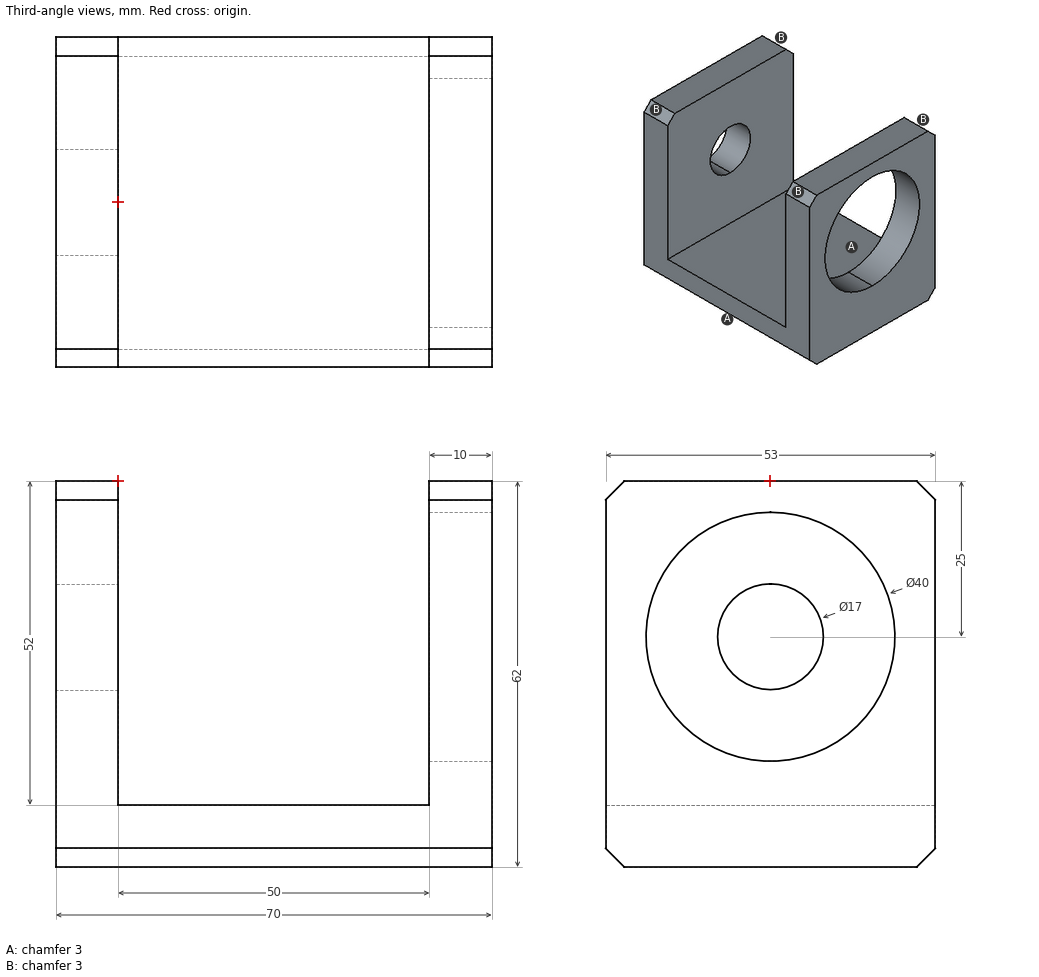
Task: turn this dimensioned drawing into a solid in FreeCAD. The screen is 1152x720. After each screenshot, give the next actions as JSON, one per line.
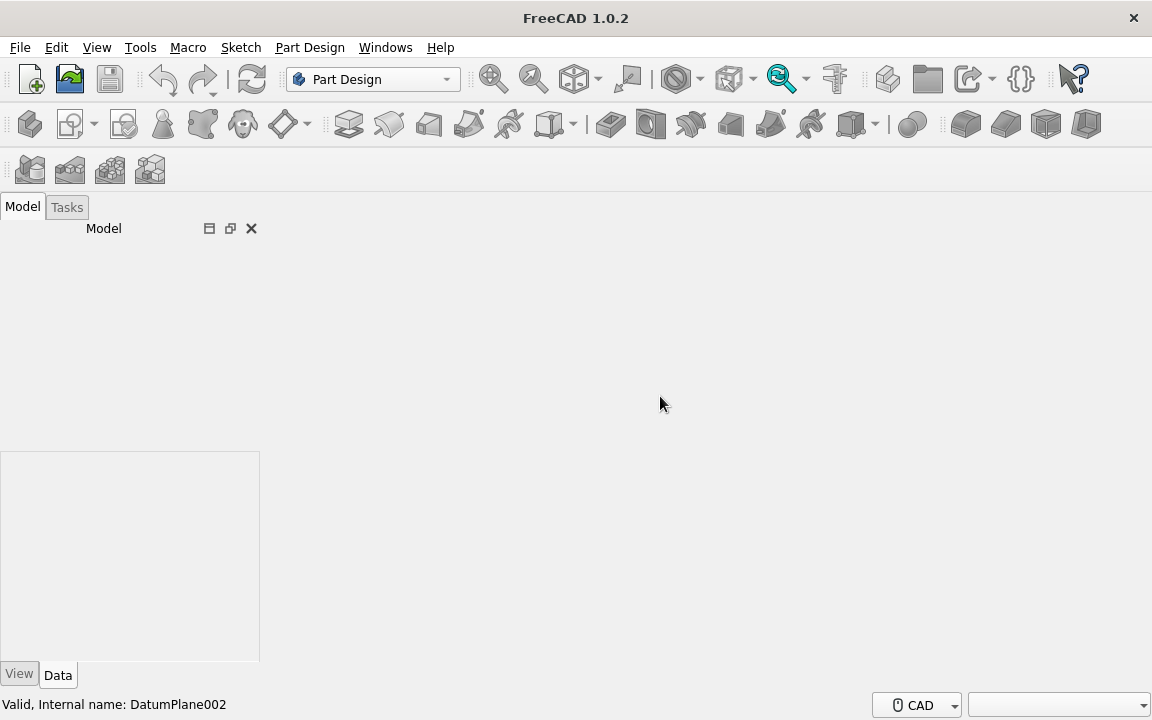
{"action": "key", "text": "ctrl+n"}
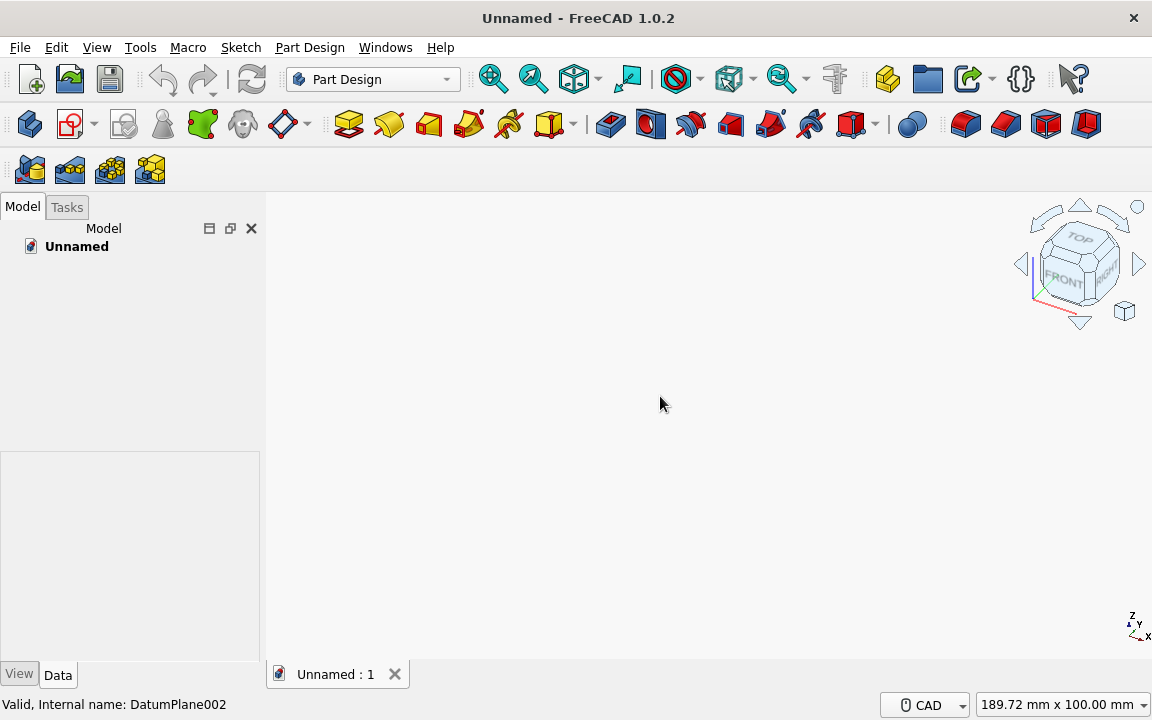
{"action": "left_click", "coordinate": [70, 124]}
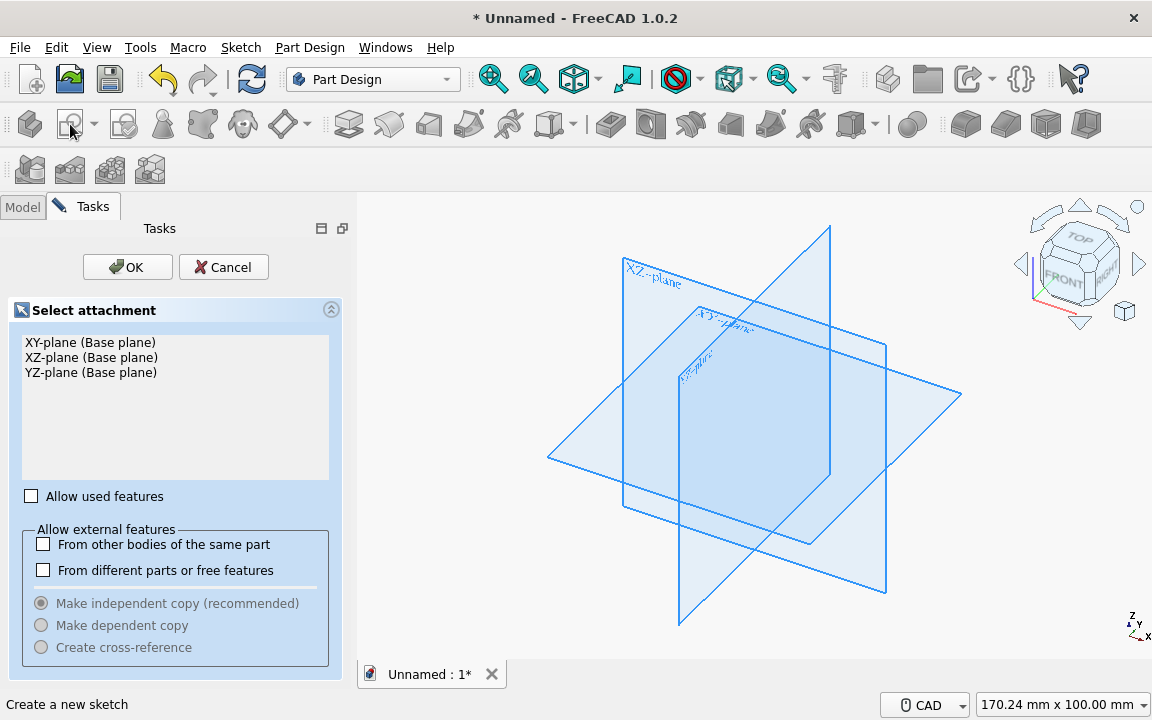
{"action": "left_click", "coordinate": [82, 358]}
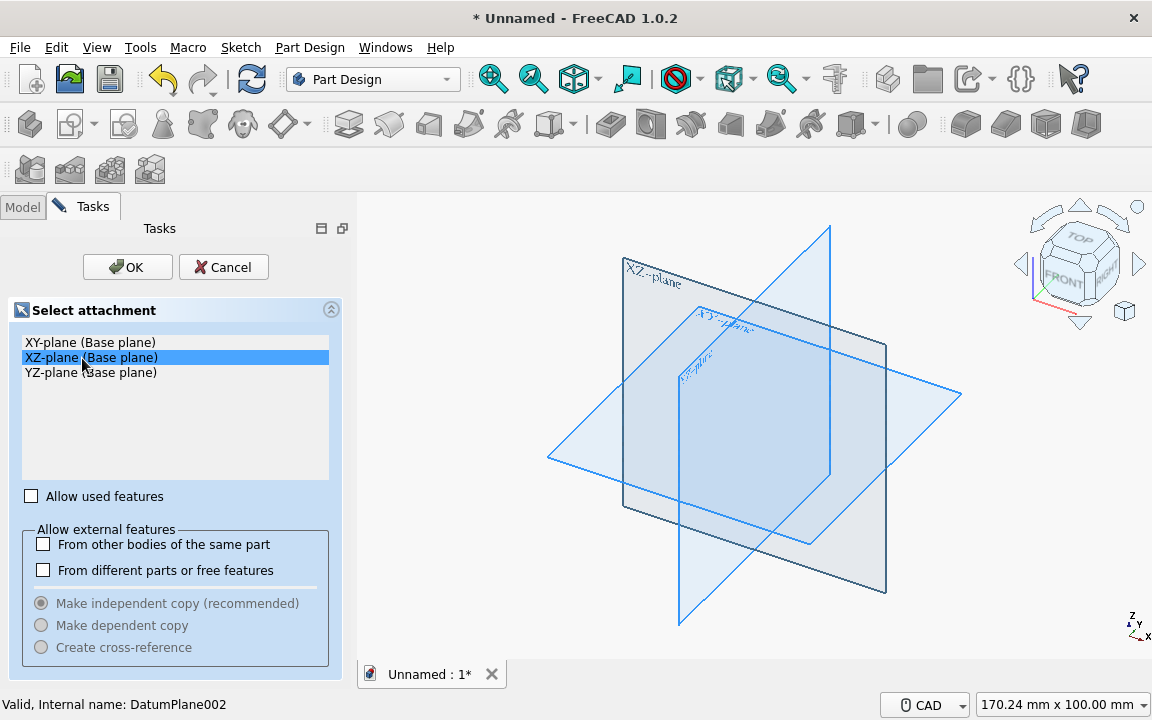
{"action": "left_click", "coordinate": [128, 267]}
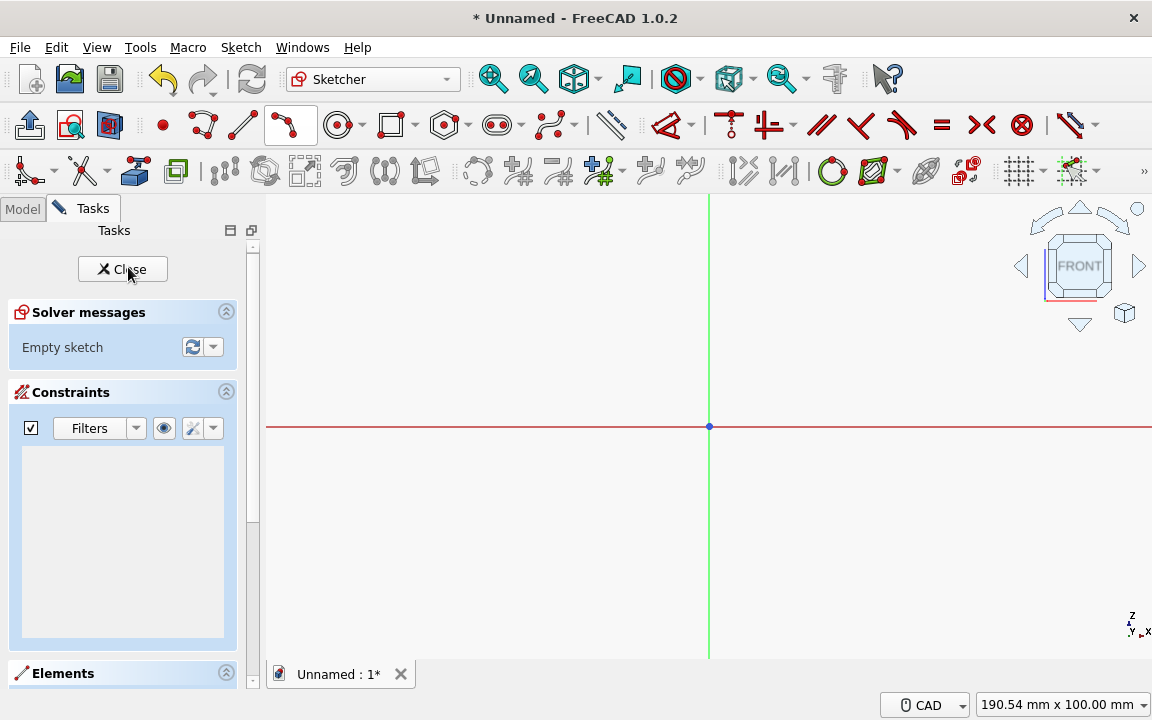
{"action": "scroll", "coordinate": [294, 222], "scroll_direction": "down", "scroll_amount": 2}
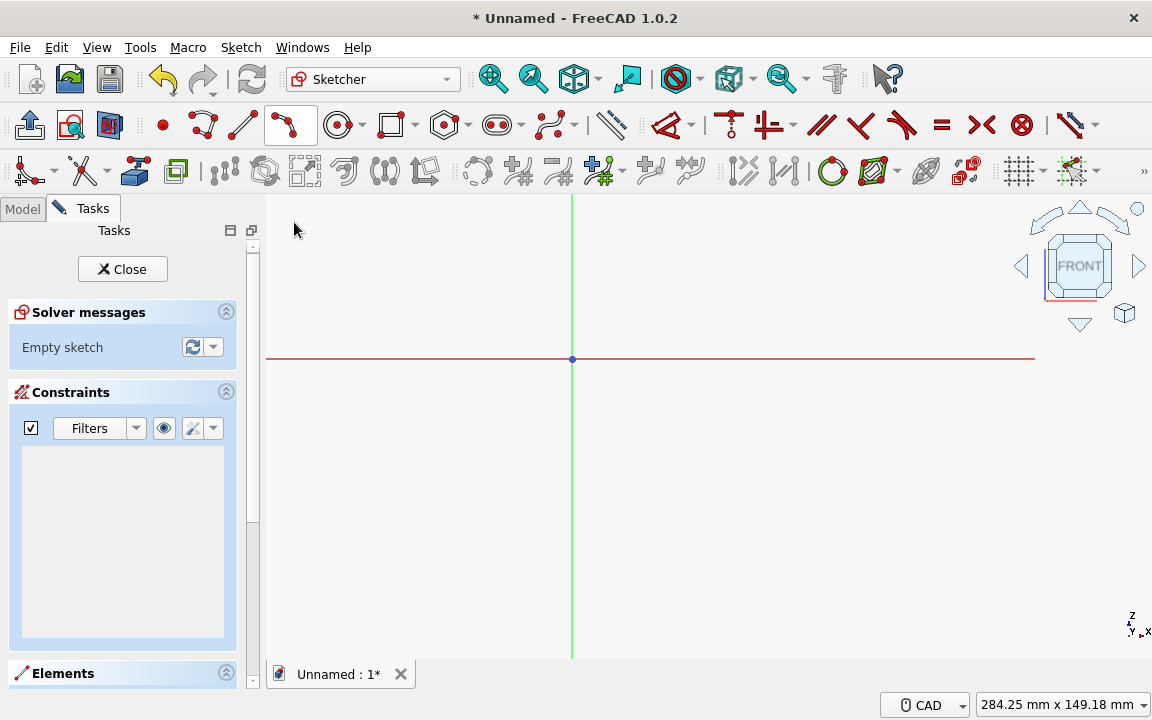
{"action": "scroll", "coordinate": [670, 515], "scroll_direction": "up", "scroll_amount": 2}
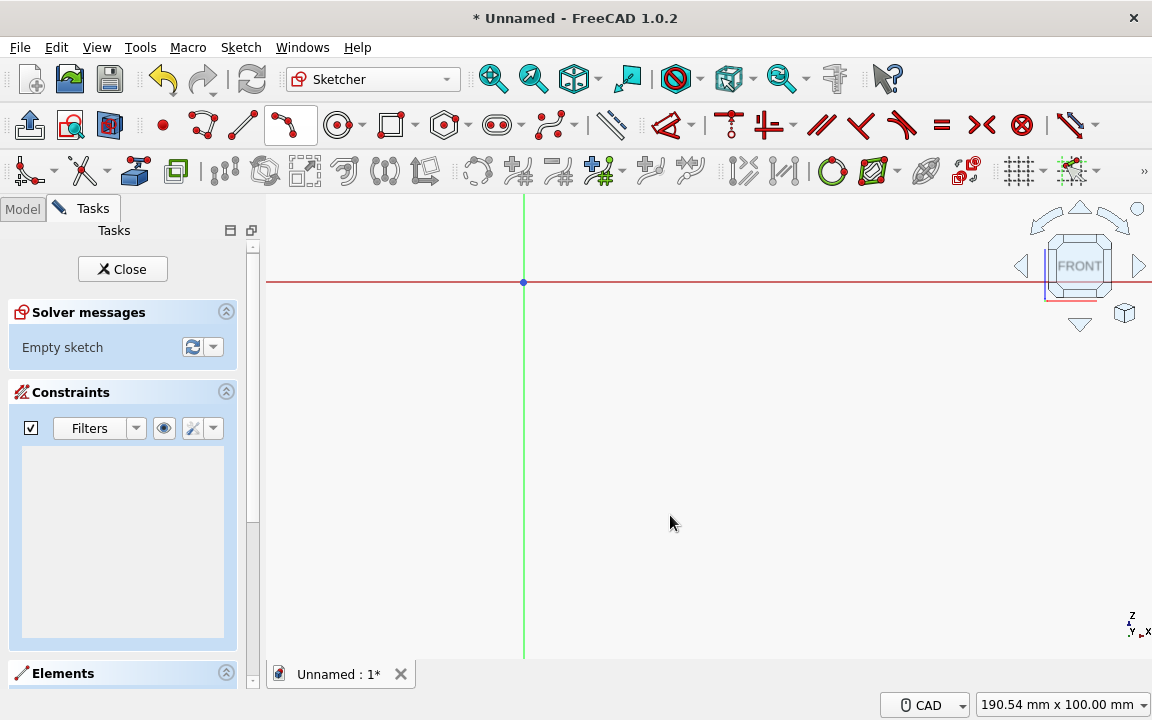
{"action": "key", "text": "g m"}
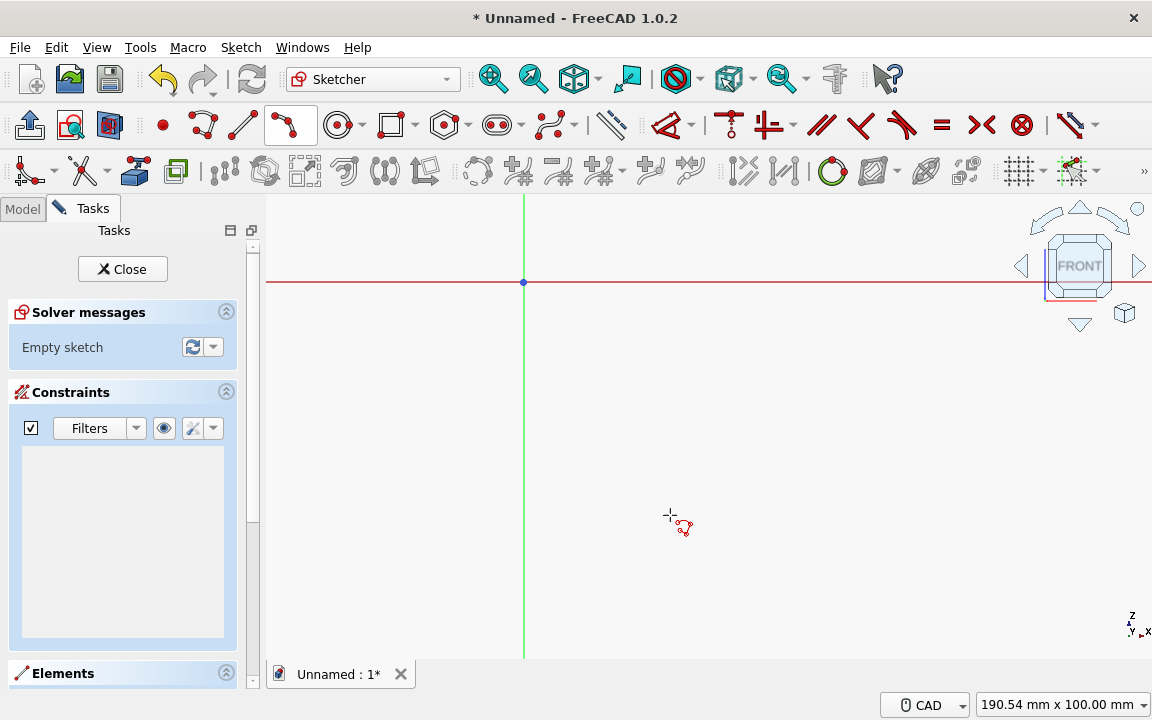
{"action": "left_click", "coordinate": [524, 282]}
{"action": "left_click", "coordinate": [533, 524]}
{"action": "left_click", "coordinate": [756, 524]}
{"action": "left_click", "coordinate": [756, 282]}
{"action": "left_click", "coordinate": [803, 291]}
{"action": "left_click", "coordinate": [803, 570]}
{"action": "left_click", "coordinate": [477, 570]}
{"action": "left_click", "coordinate": [477, 291]}
{"action": "left_click", "coordinate": [524, 282]}
{"action": "key", "text": "Escape"}
{"action": "key", "text": "Escape"}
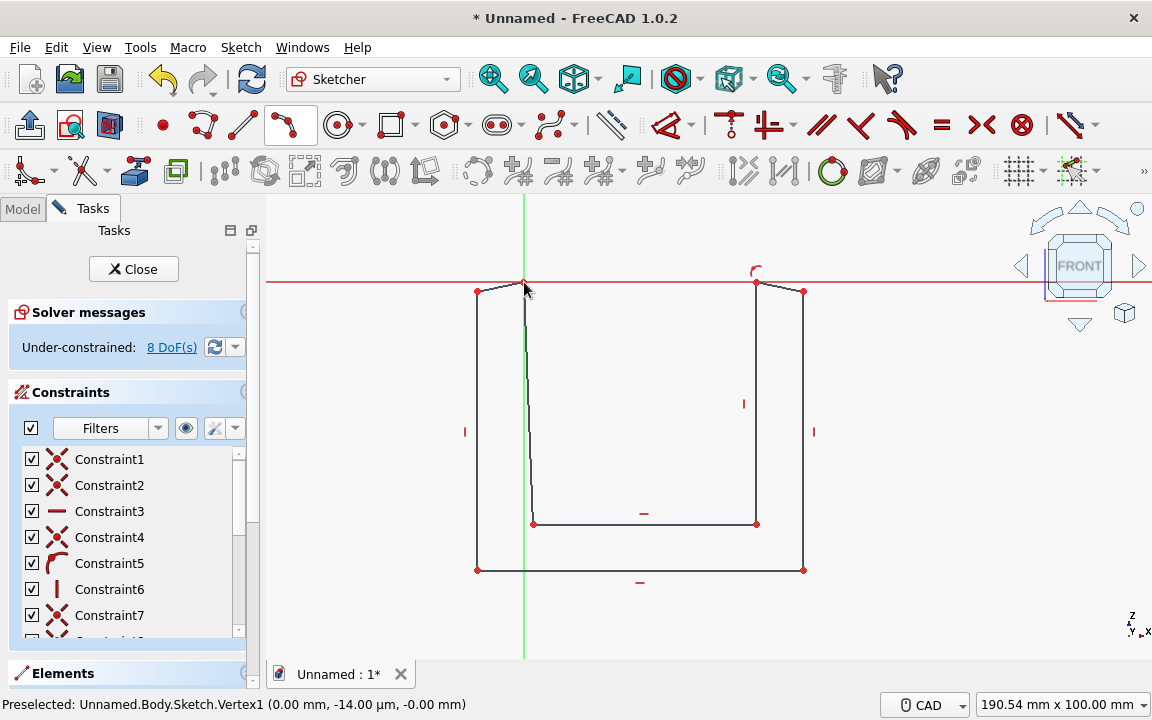
{"action": "left_click", "coordinate": [527, 355]}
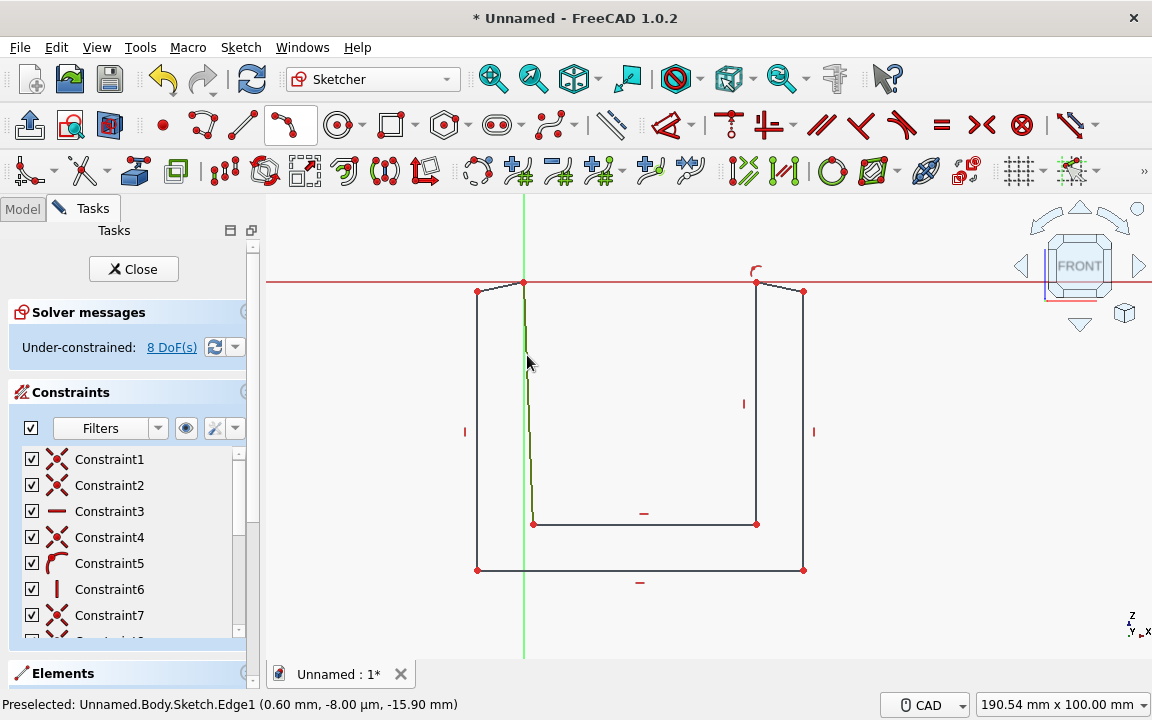
{"action": "left_click", "coordinate": [796, 126]}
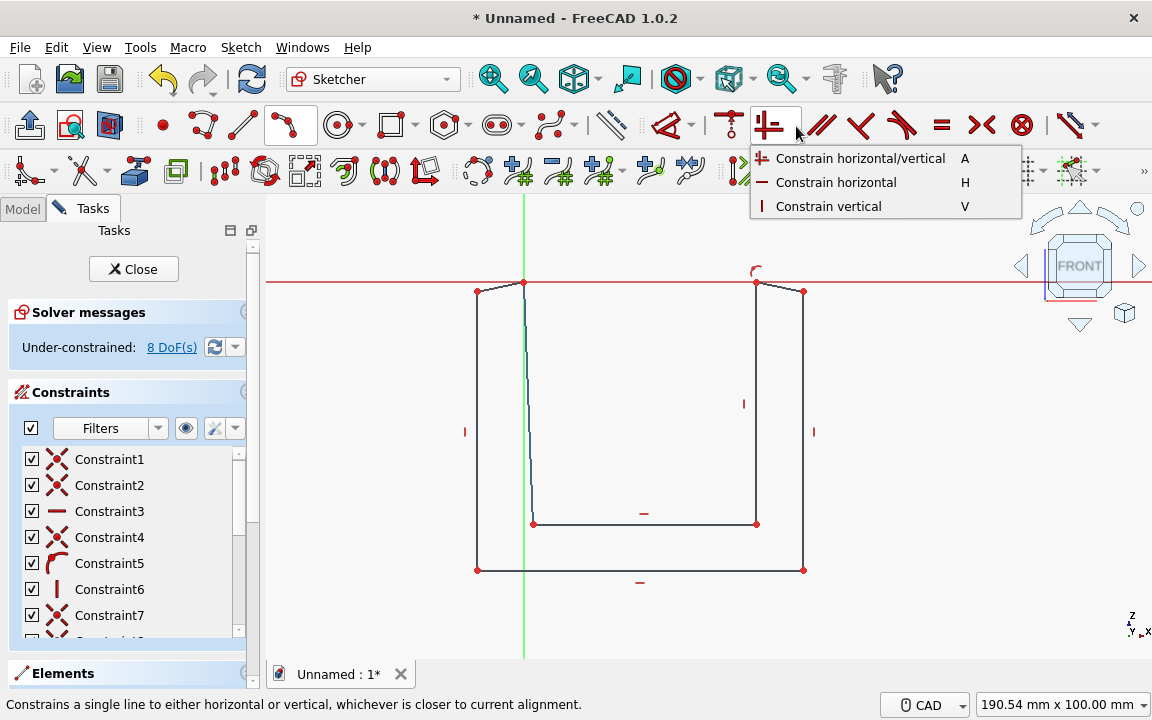
{"action": "left_click", "coordinate": [886, 206]}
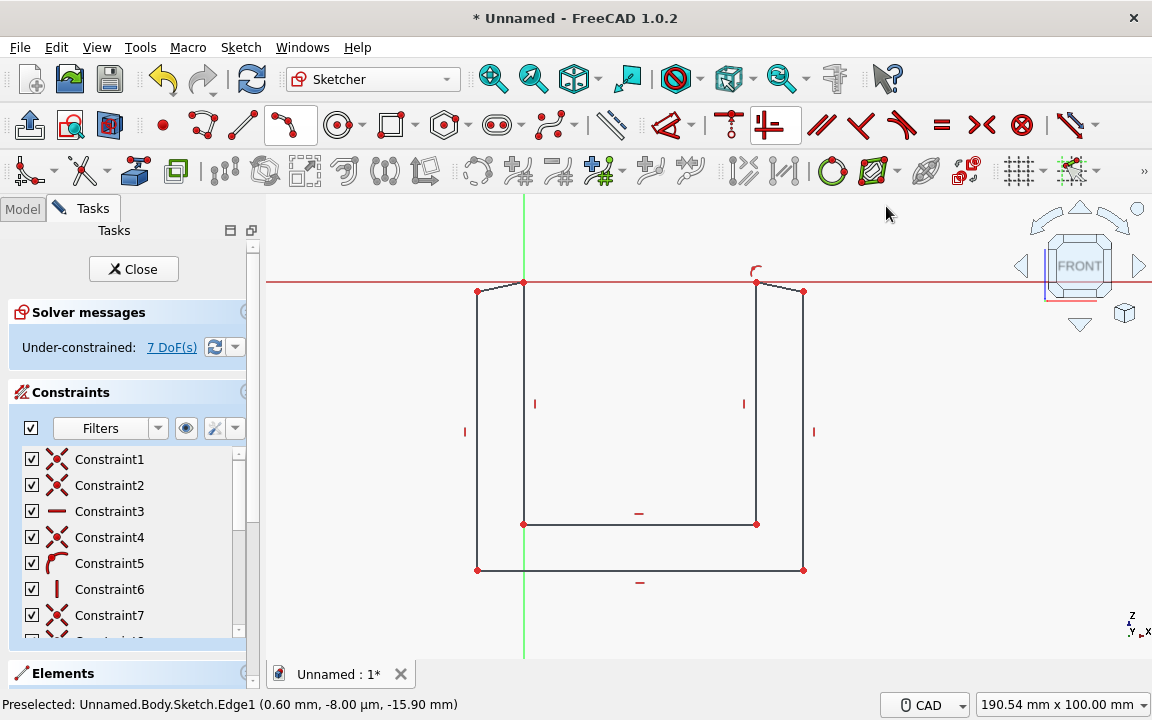
{"action": "left_click", "coordinate": [770, 285]}